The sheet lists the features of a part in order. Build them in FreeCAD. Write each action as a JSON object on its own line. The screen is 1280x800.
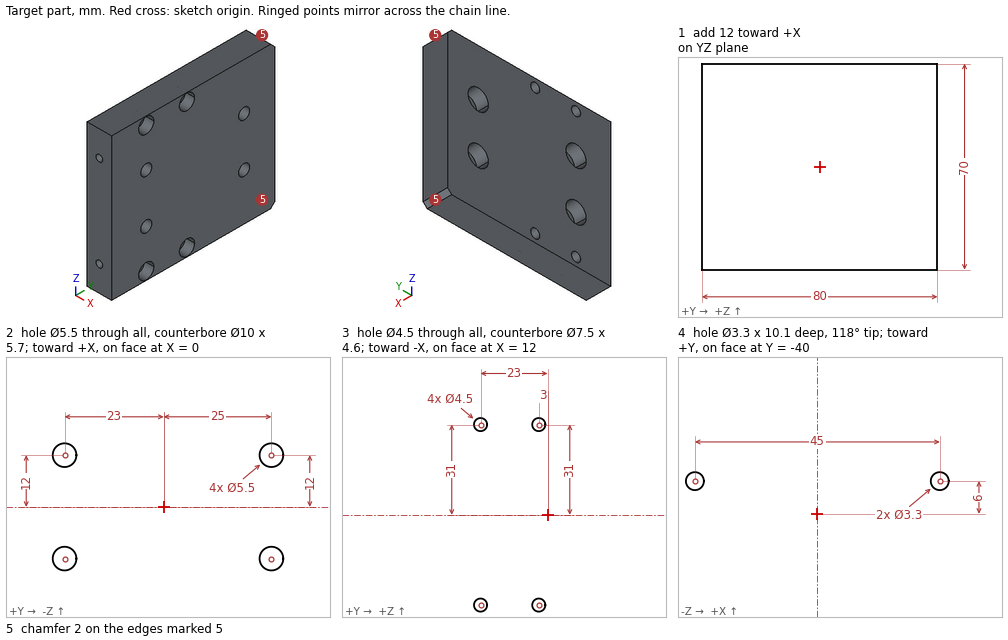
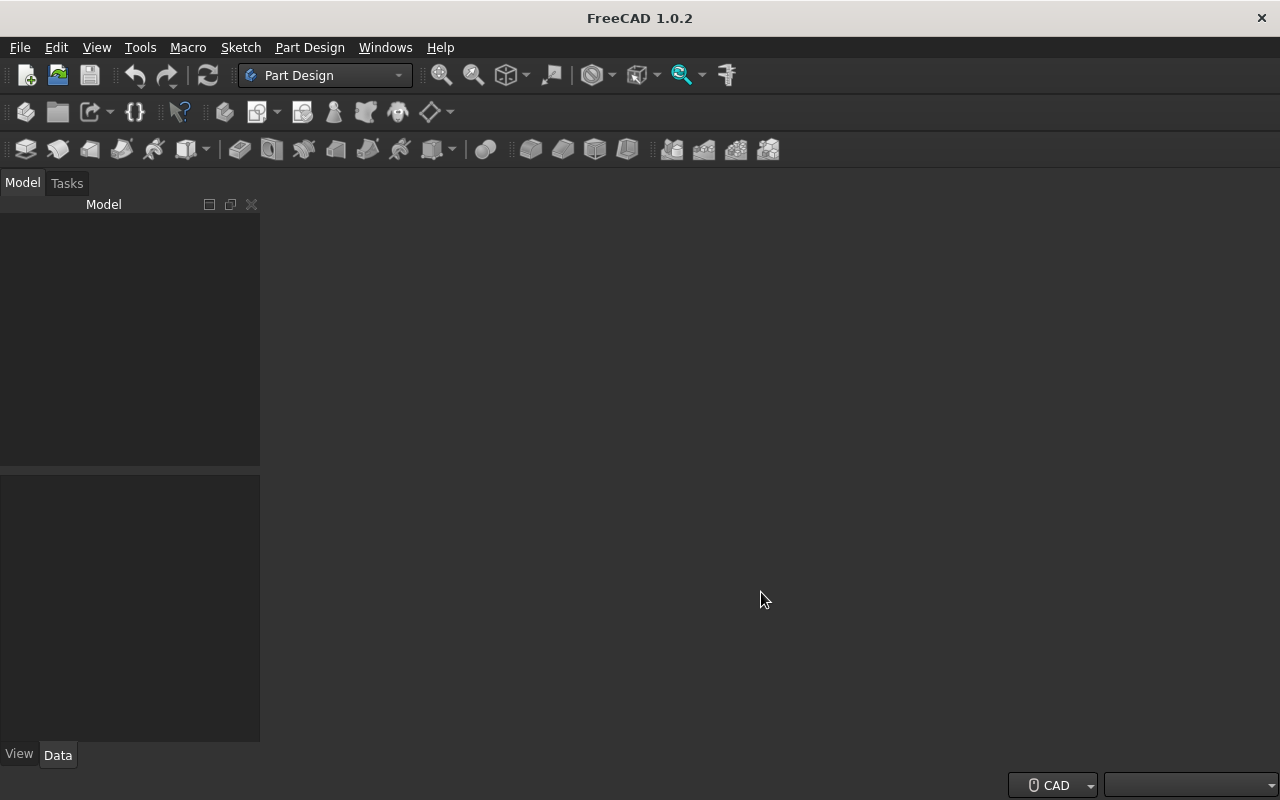
{"action": "left_click", "coordinate": [26, 76]}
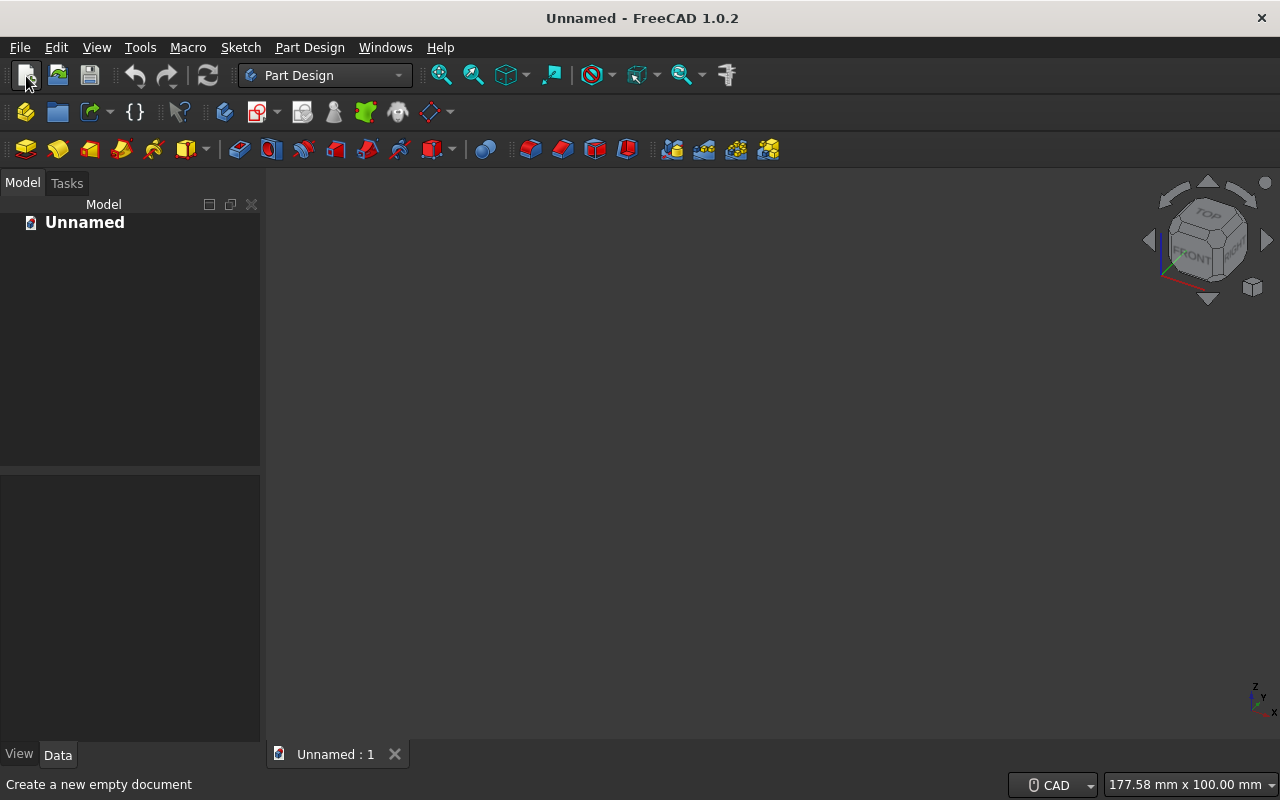
{"action": "left_click", "coordinate": [258, 112]}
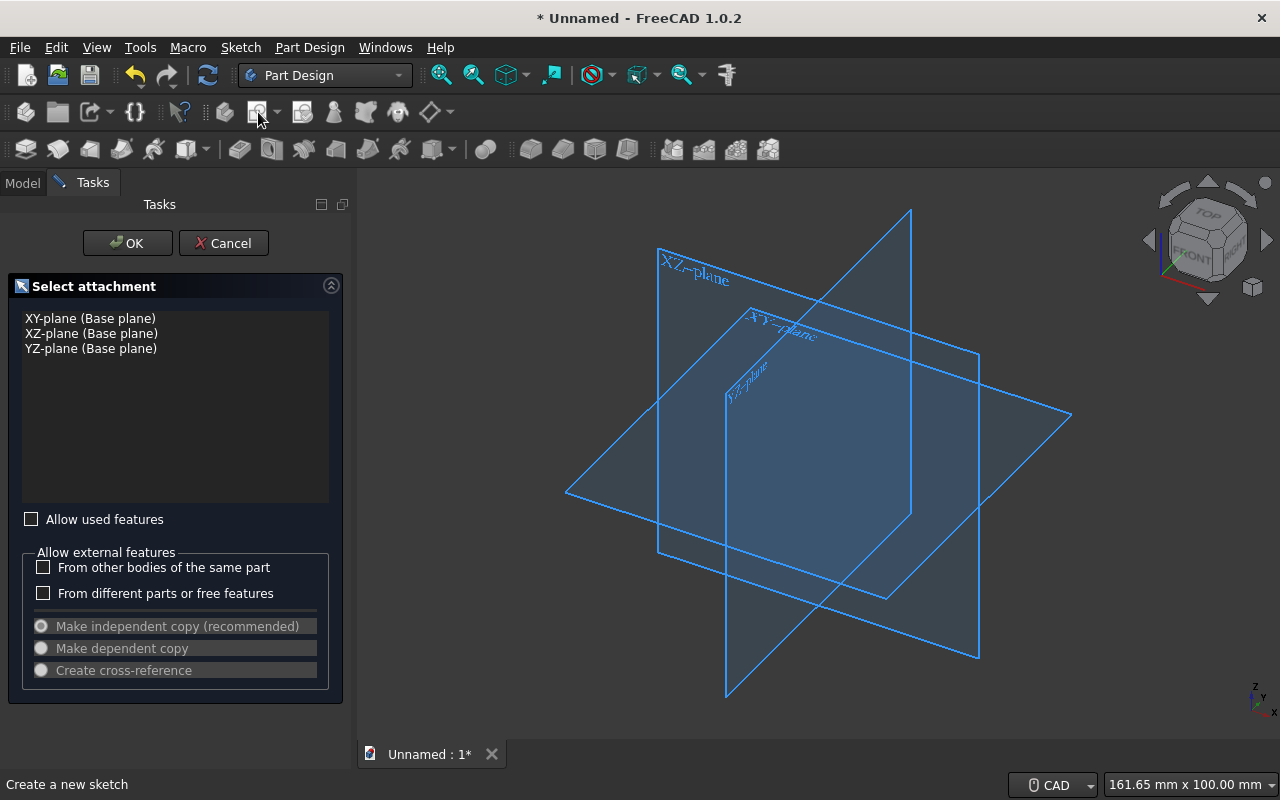
{"action": "left_click", "coordinate": [82, 348]}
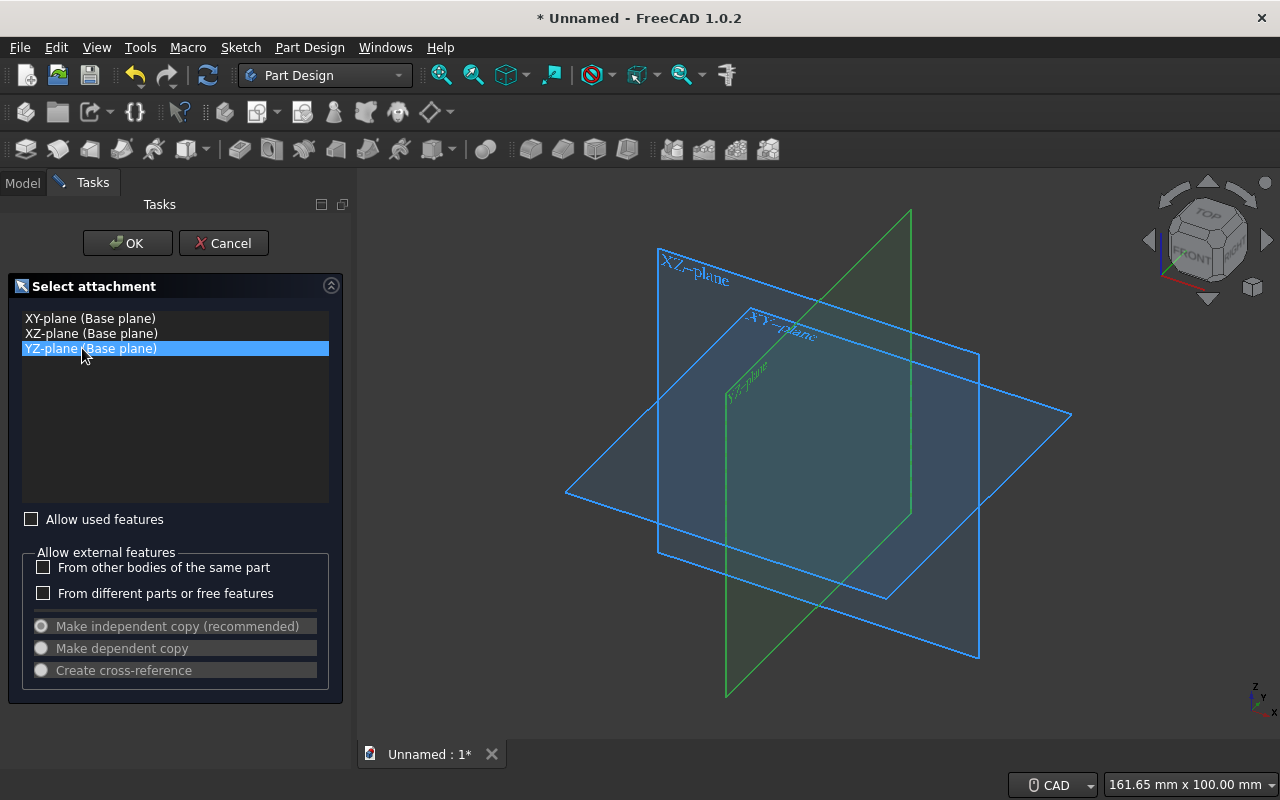
{"action": "left_click", "coordinate": [128, 243]}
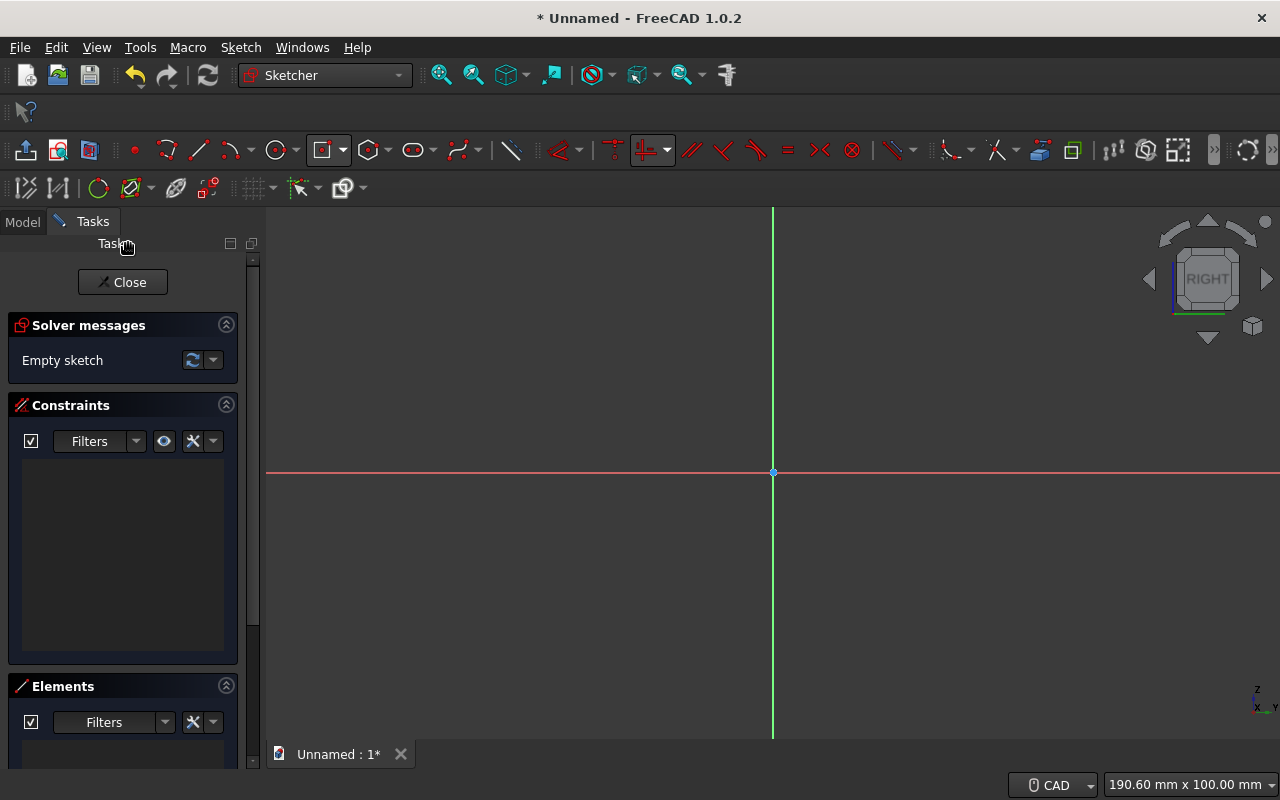
{"action": "left_click", "coordinate": [322, 150]}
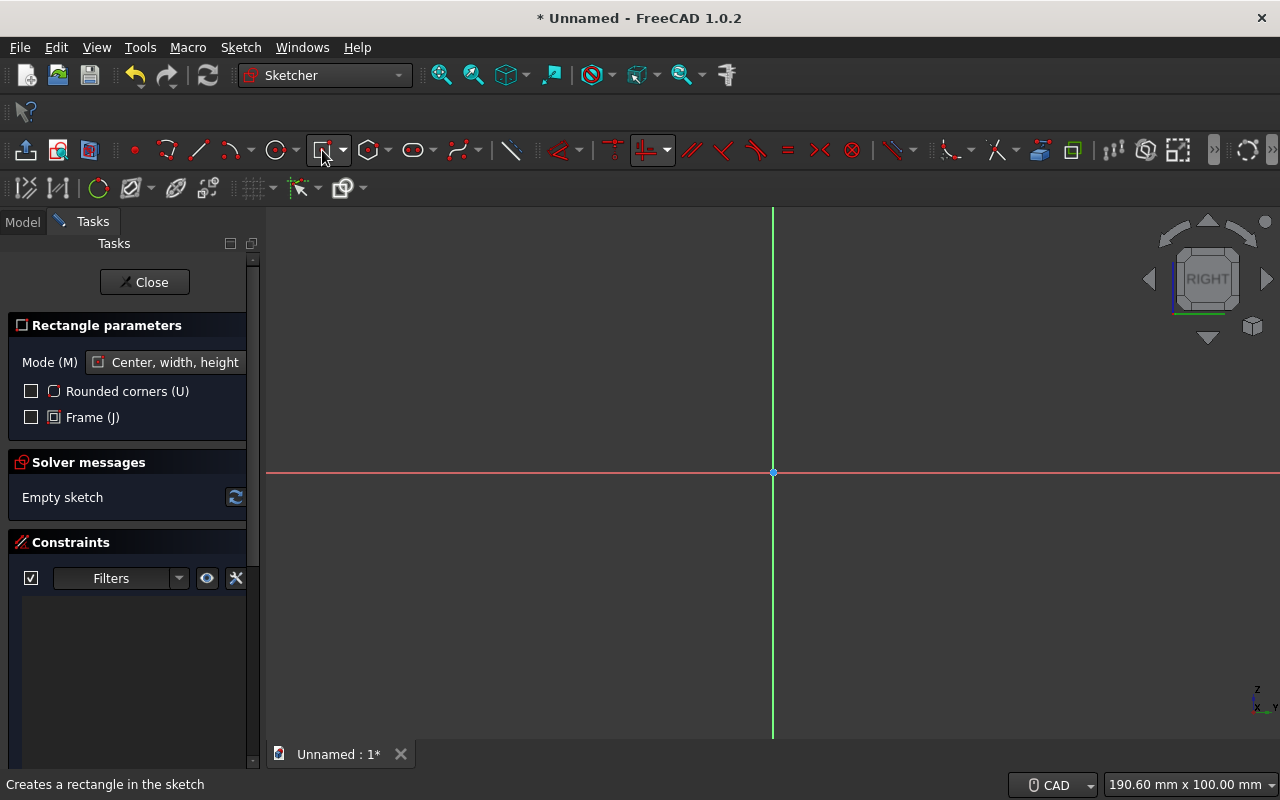
{"action": "left_click", "coordinate": [773, 473]}
{"action": "left_click", "coordinate": [986, 287]}
{"action": "key", "text": "Escape"}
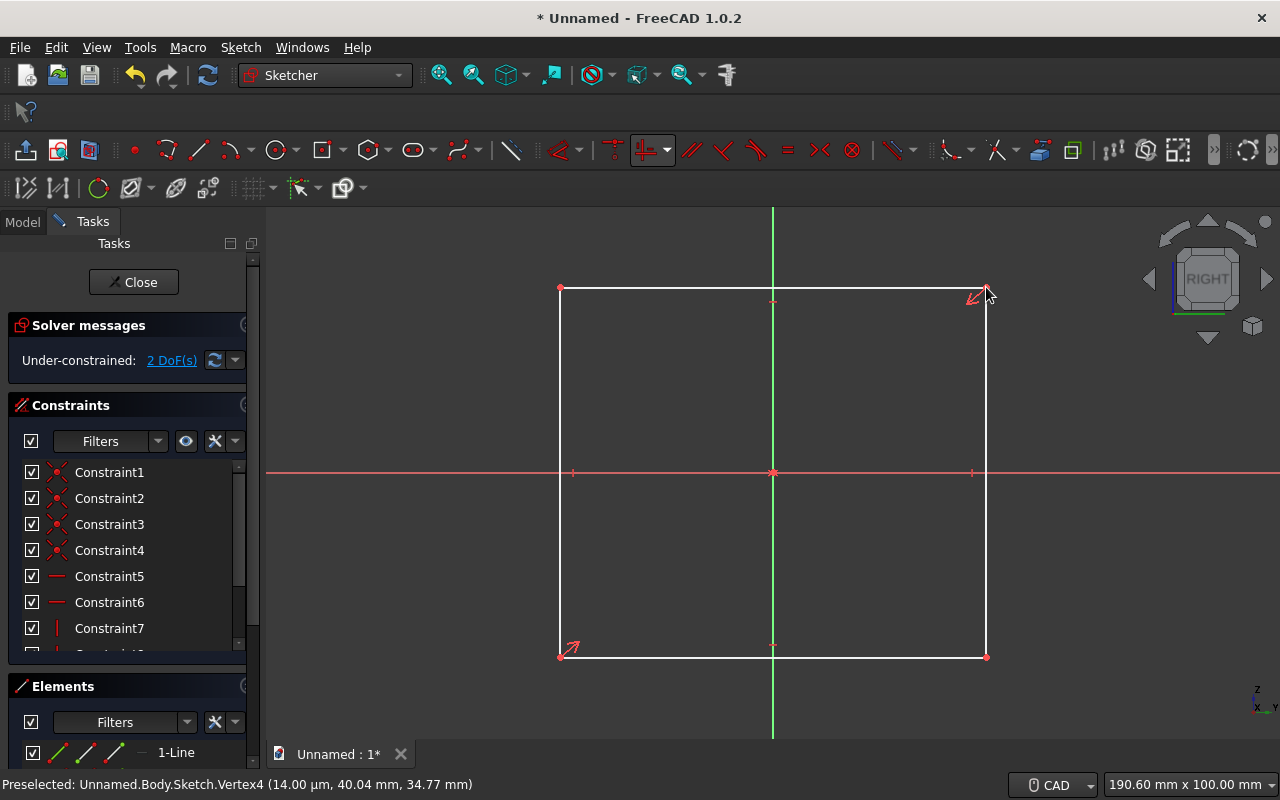
{"action": "left_click", "coordinate": [558, 150]}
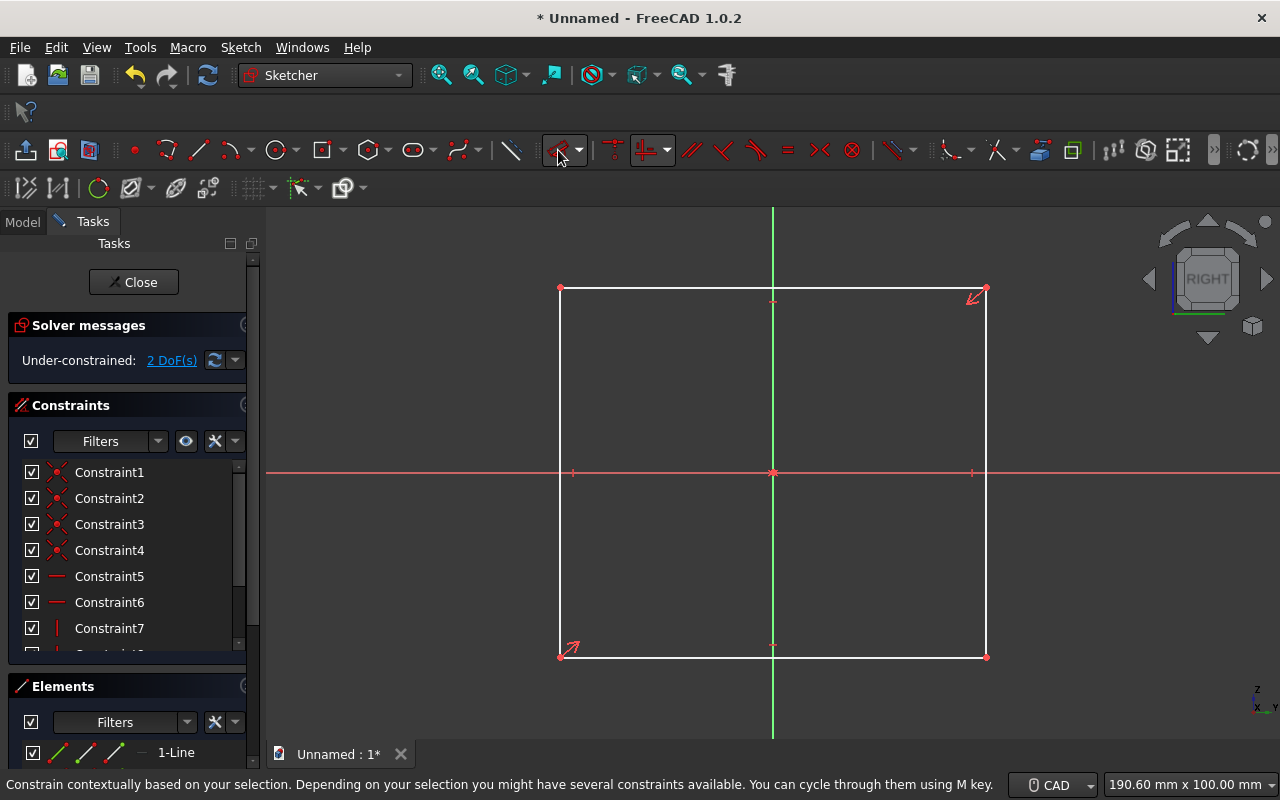
{"action": "left_click", "coordinate": [688, 658]}
{"action": "left_click", "coordinate": [675, 692]}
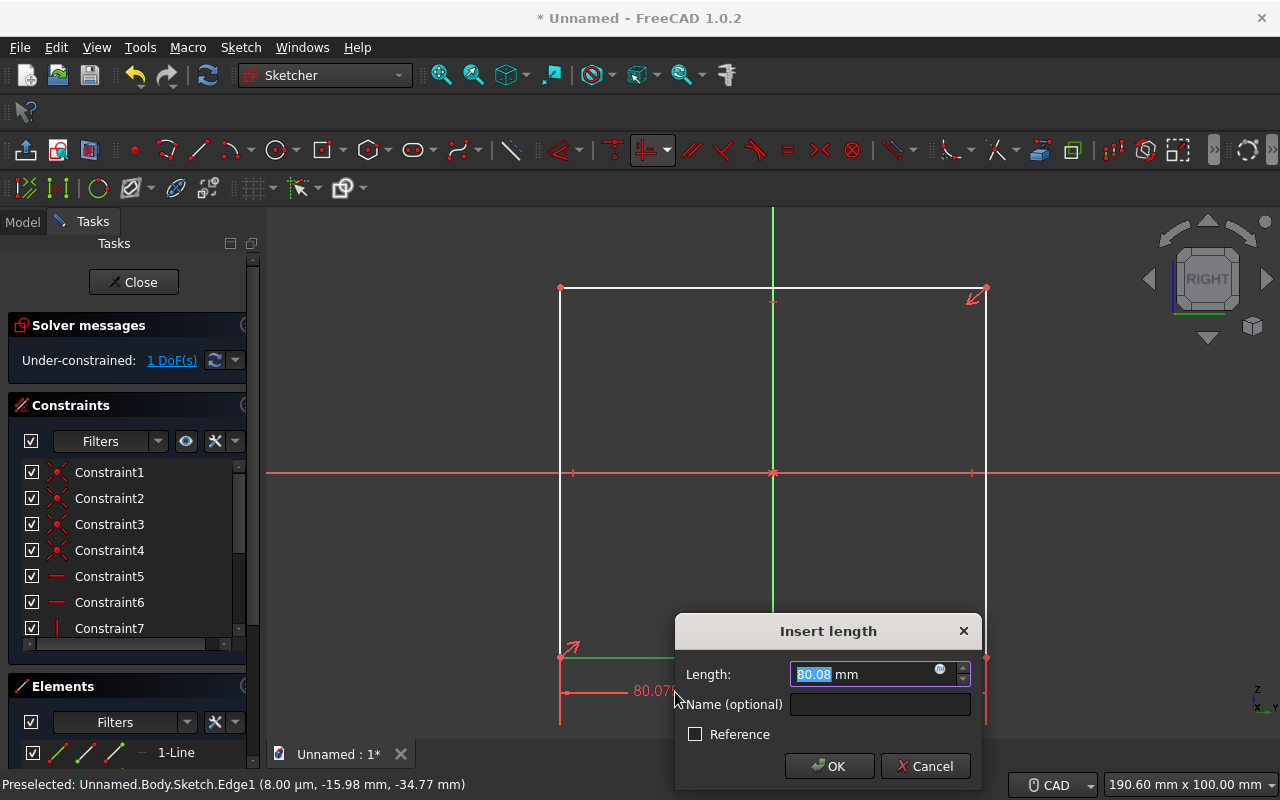
{"action": "type", "text": "80"}
{"action": "key", "text": "Return"}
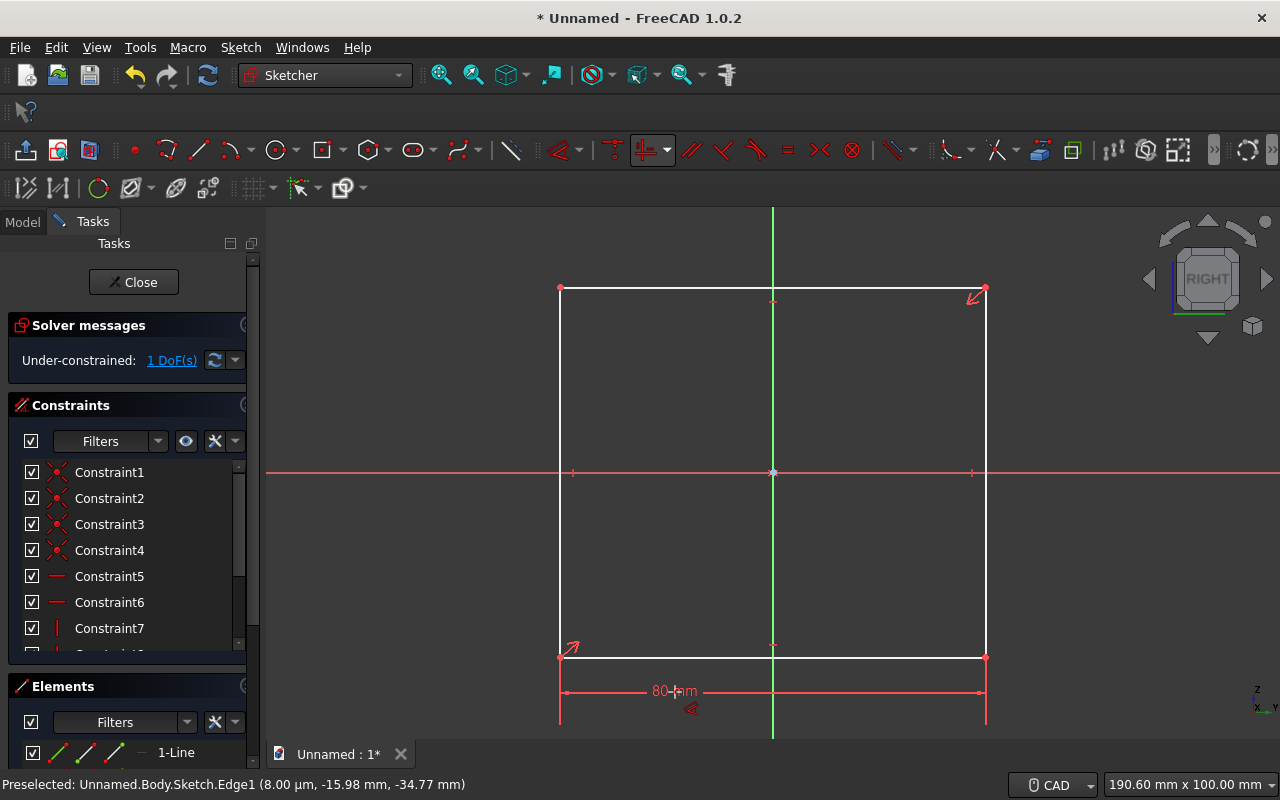
{"action": "left_click", "coordinate": [986, 547]}
{"action": "left_click", "coordinate": [1020, 388]}